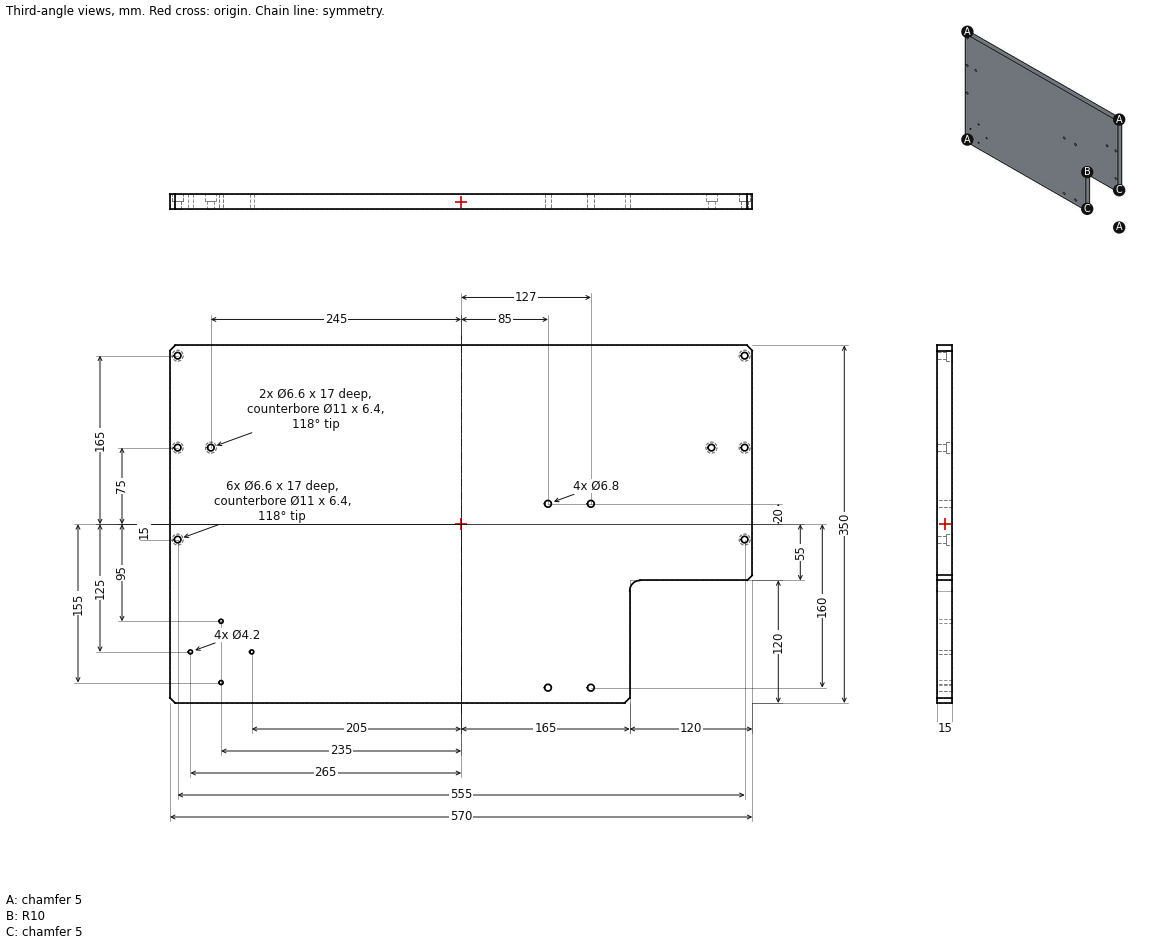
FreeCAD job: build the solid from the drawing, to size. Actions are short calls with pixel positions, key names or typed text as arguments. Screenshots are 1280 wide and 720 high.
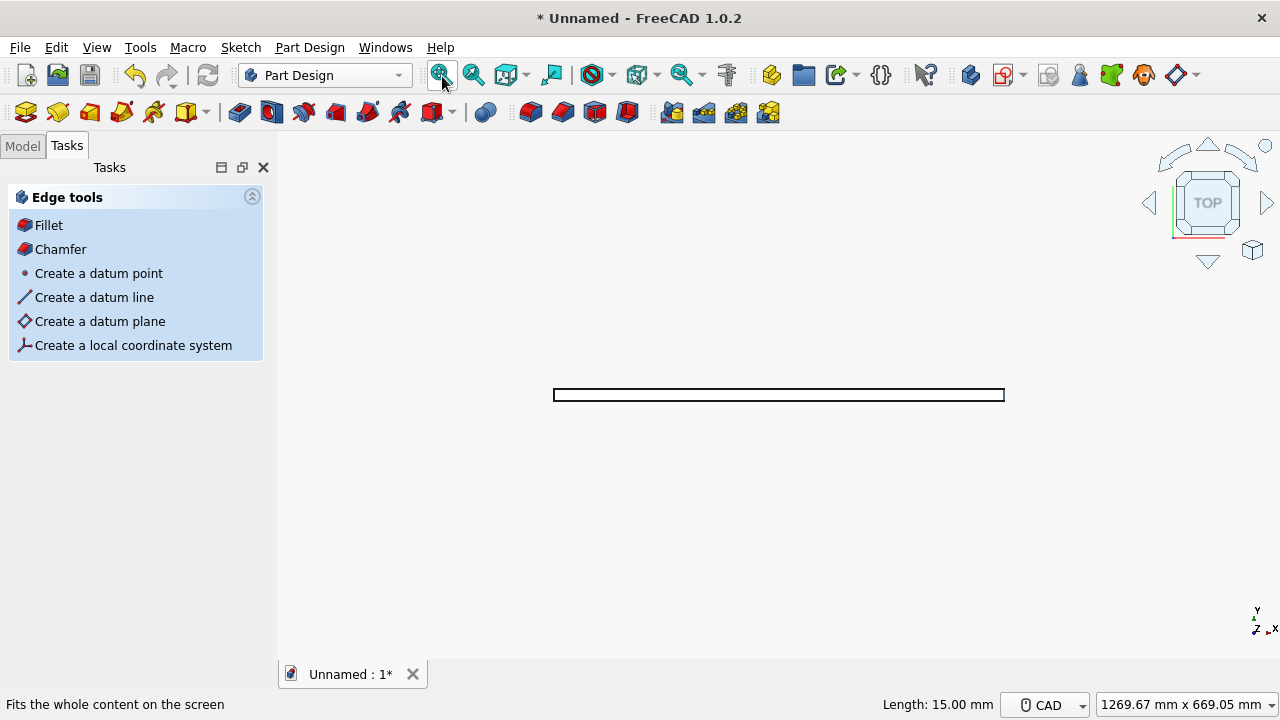
click(442, 76)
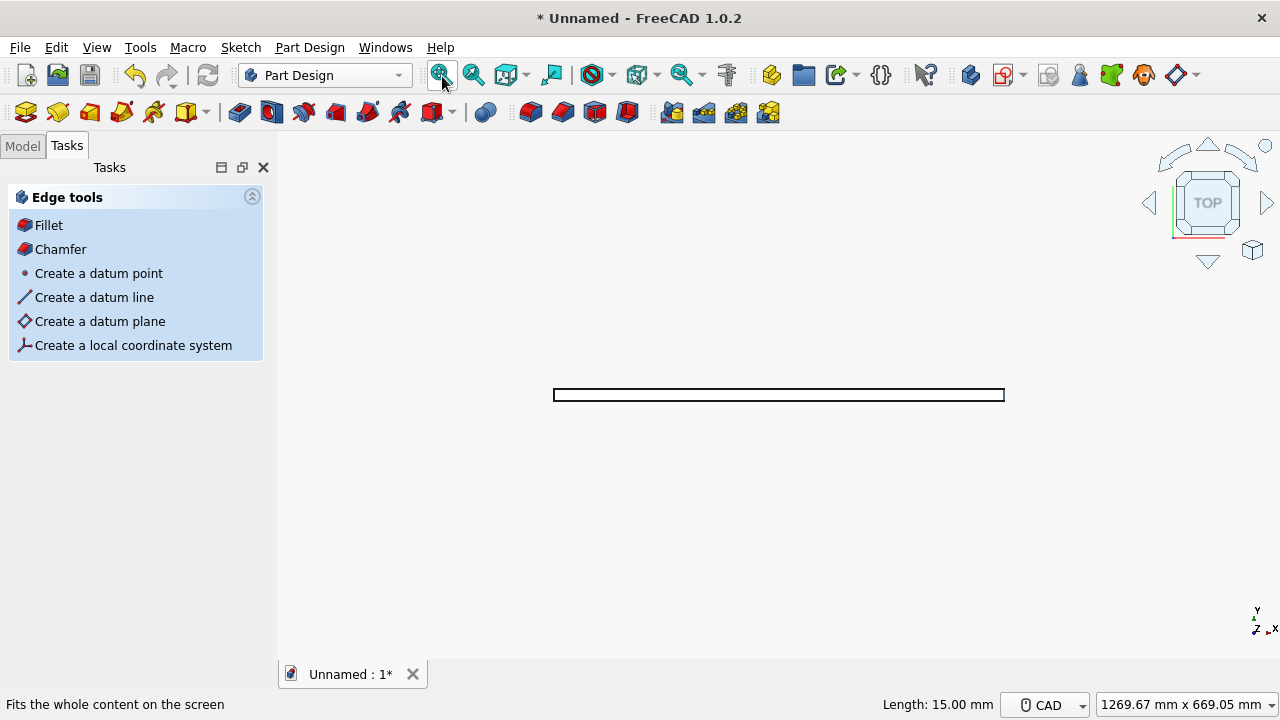
click(554, 395, ctrl)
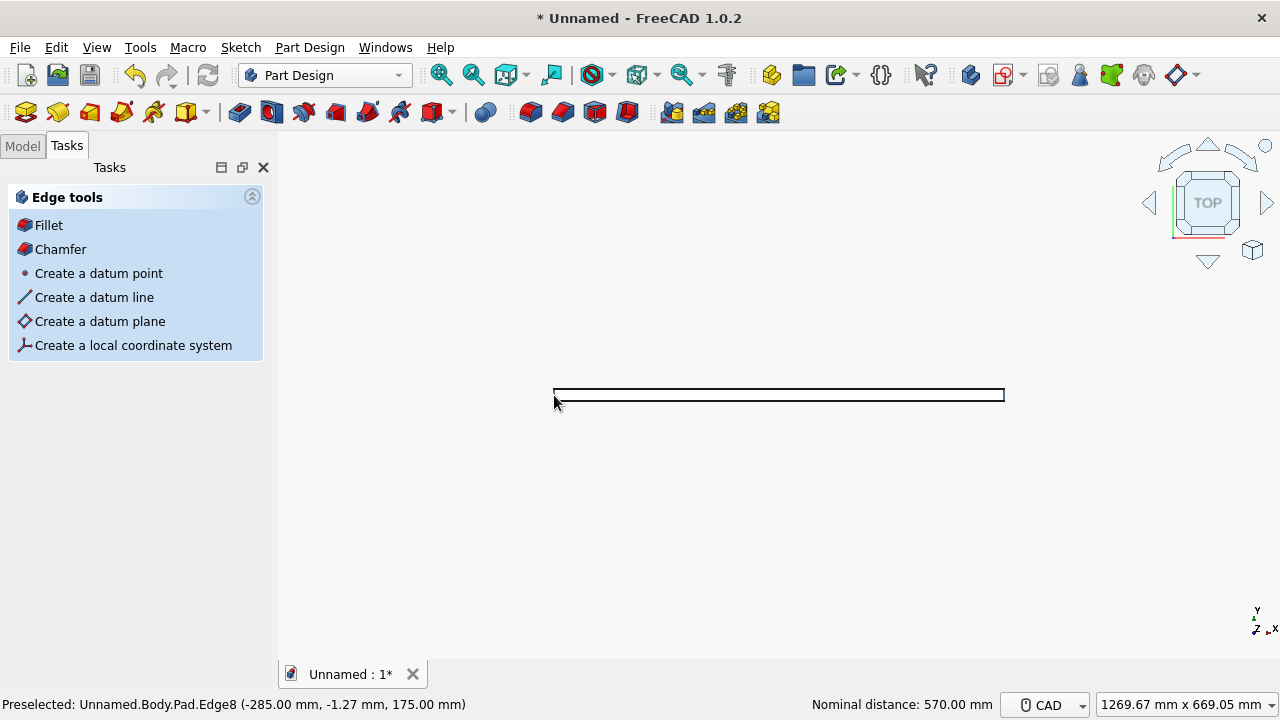
scroll(554, 394, up, 7)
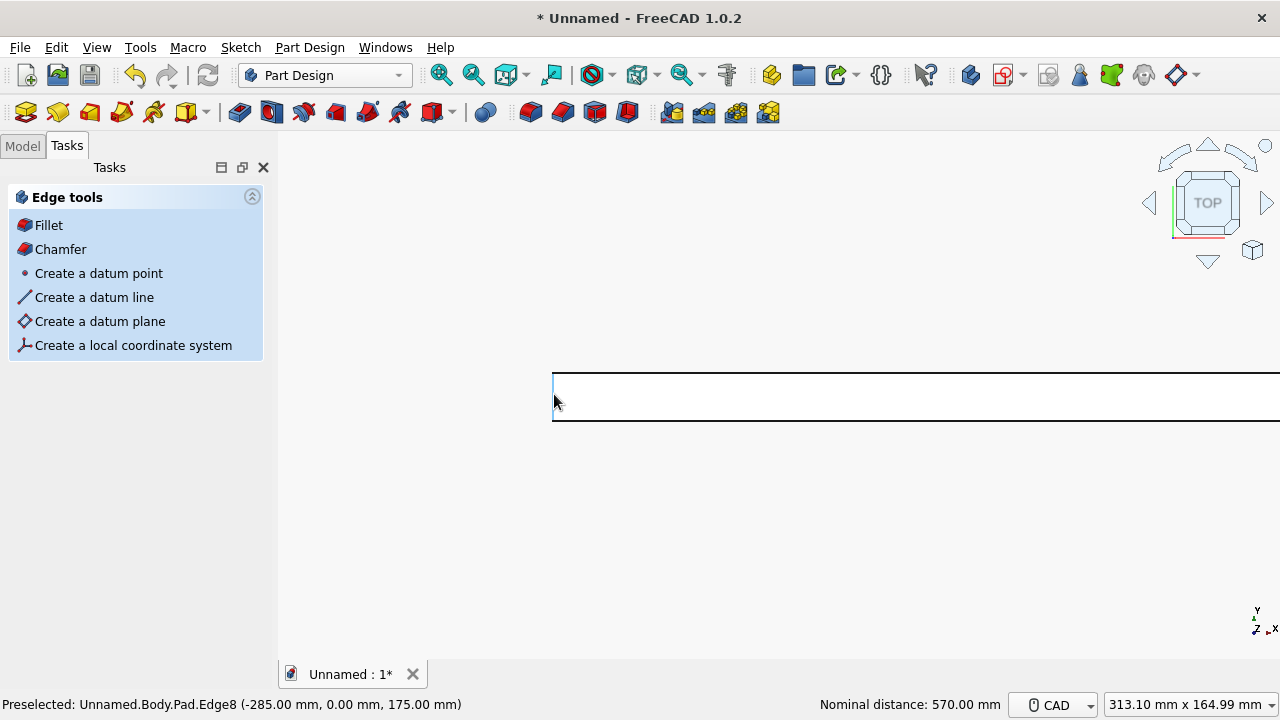
click(442, 76)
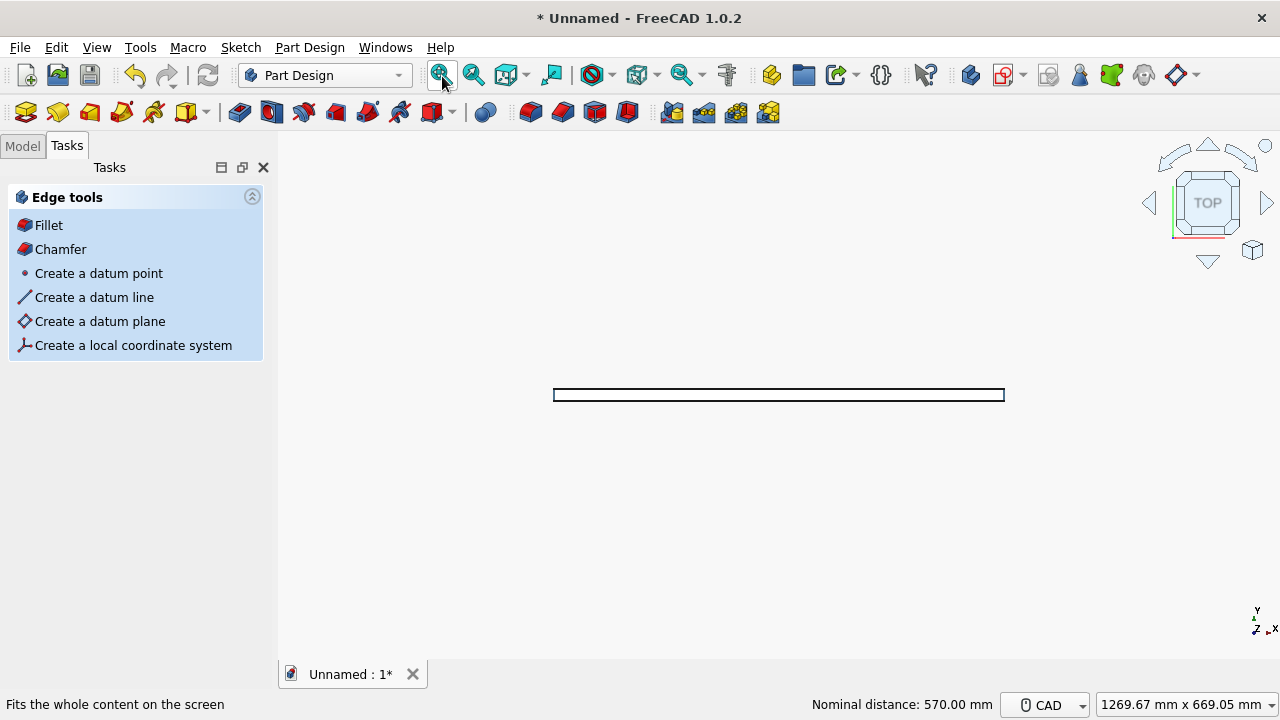
key(1)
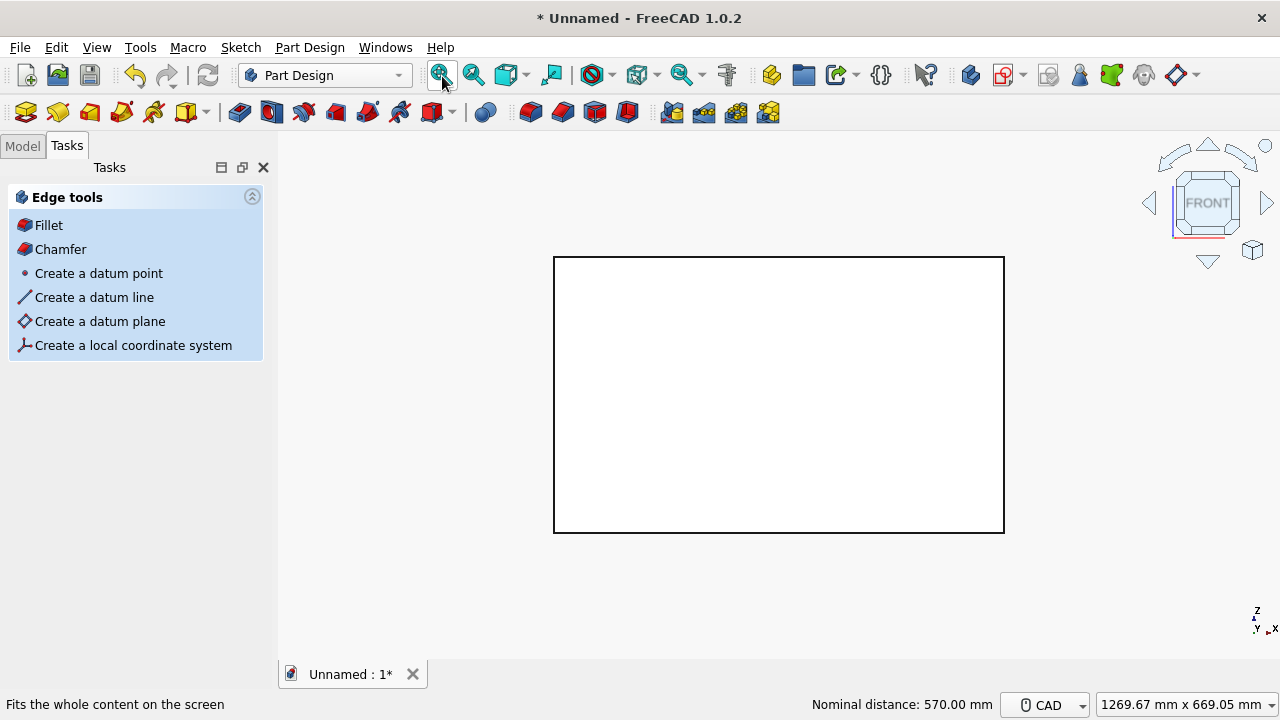
scroll(554, 532, up, 7)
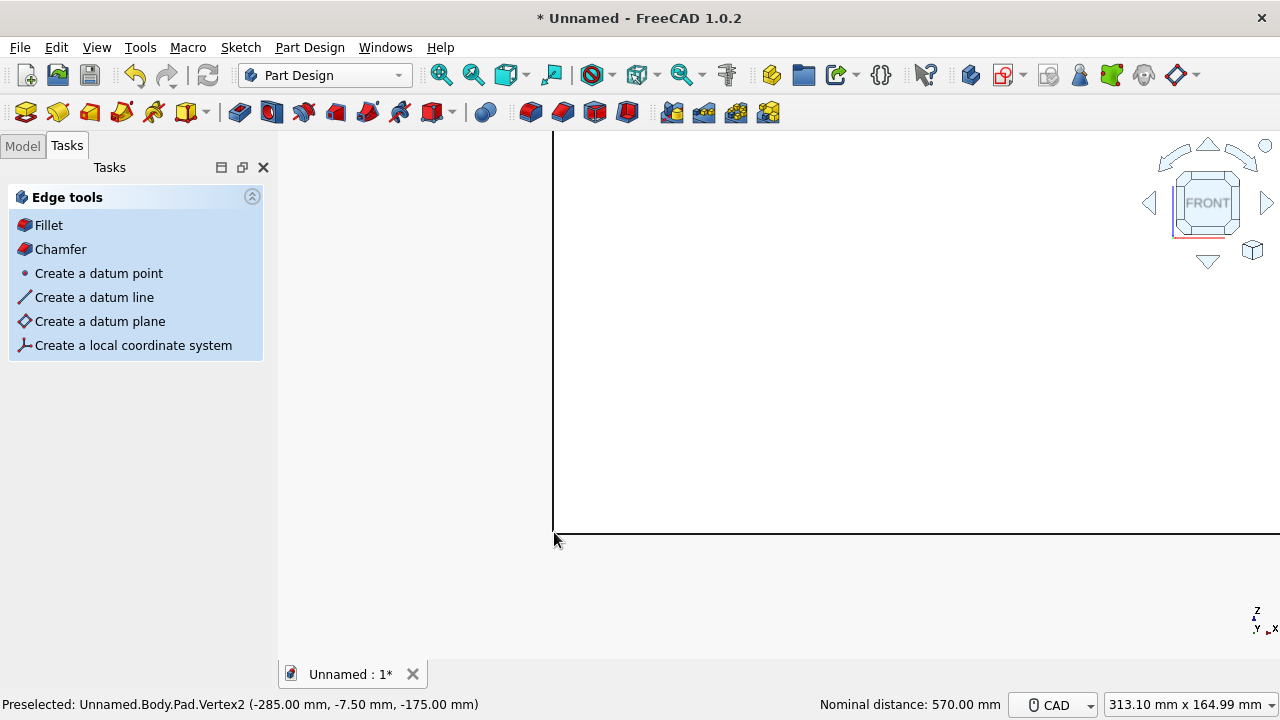
click(442, 76)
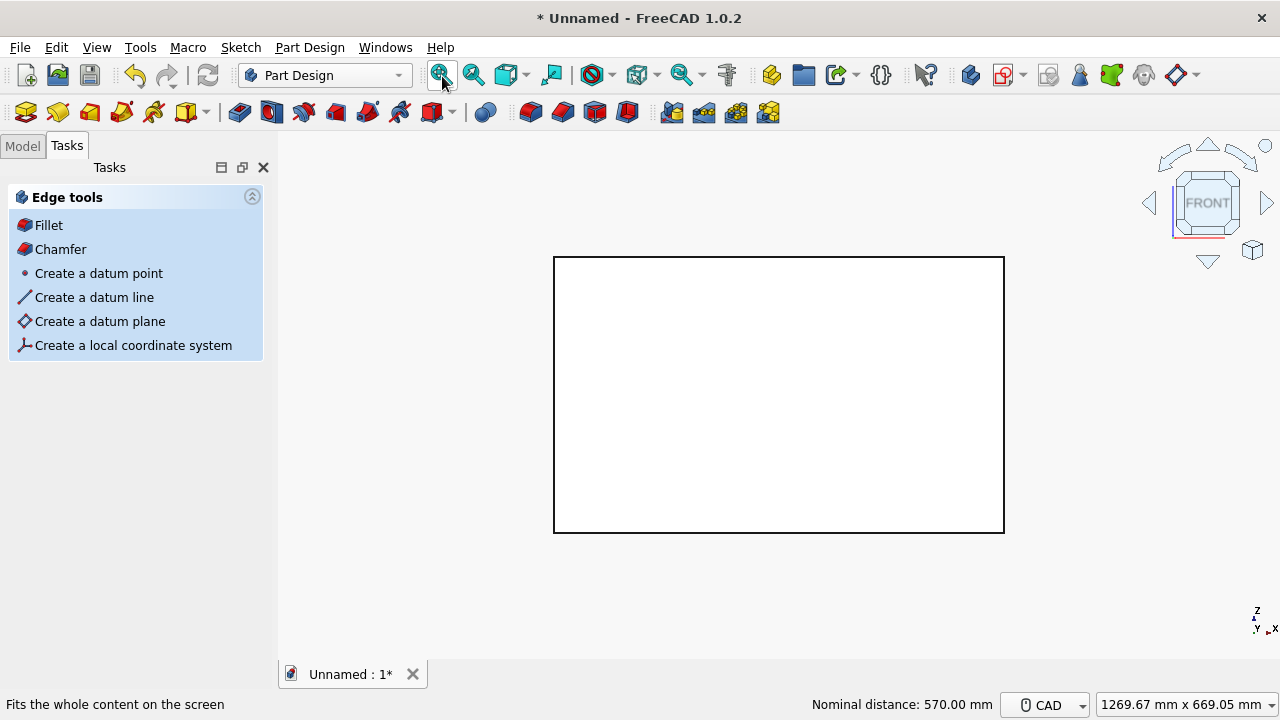
key(3)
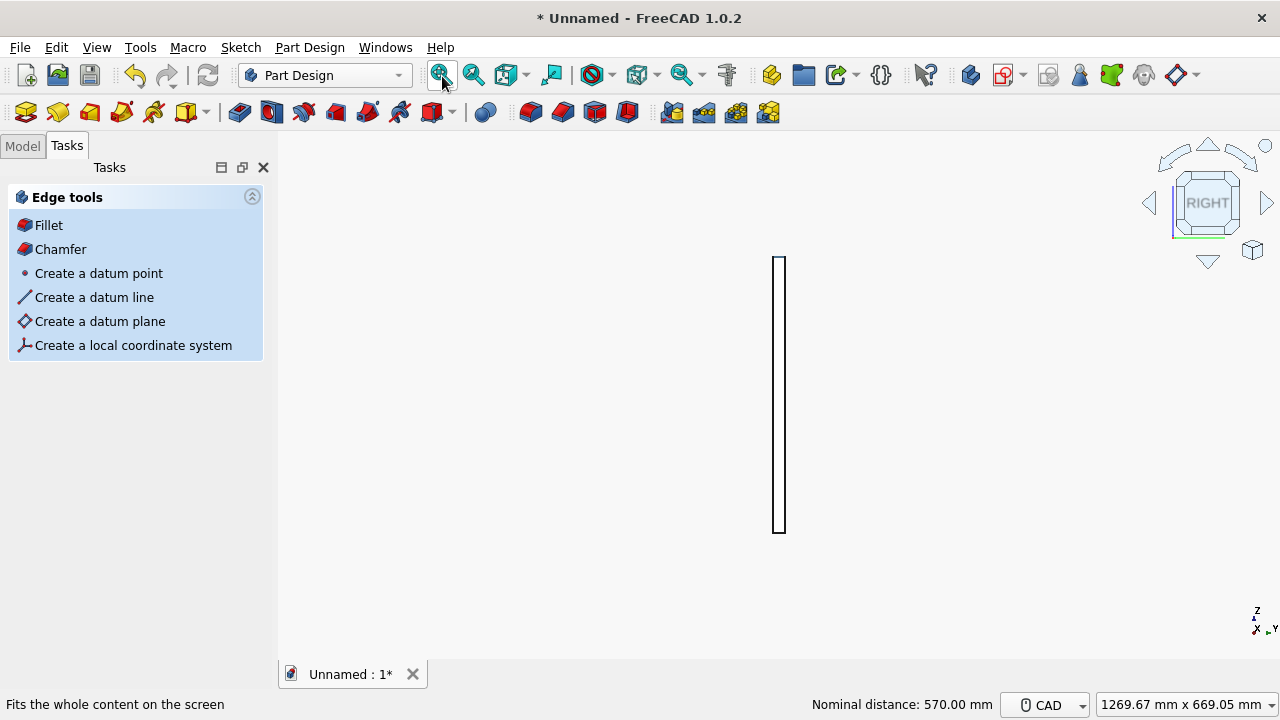
scroll(779, 532, up, 7)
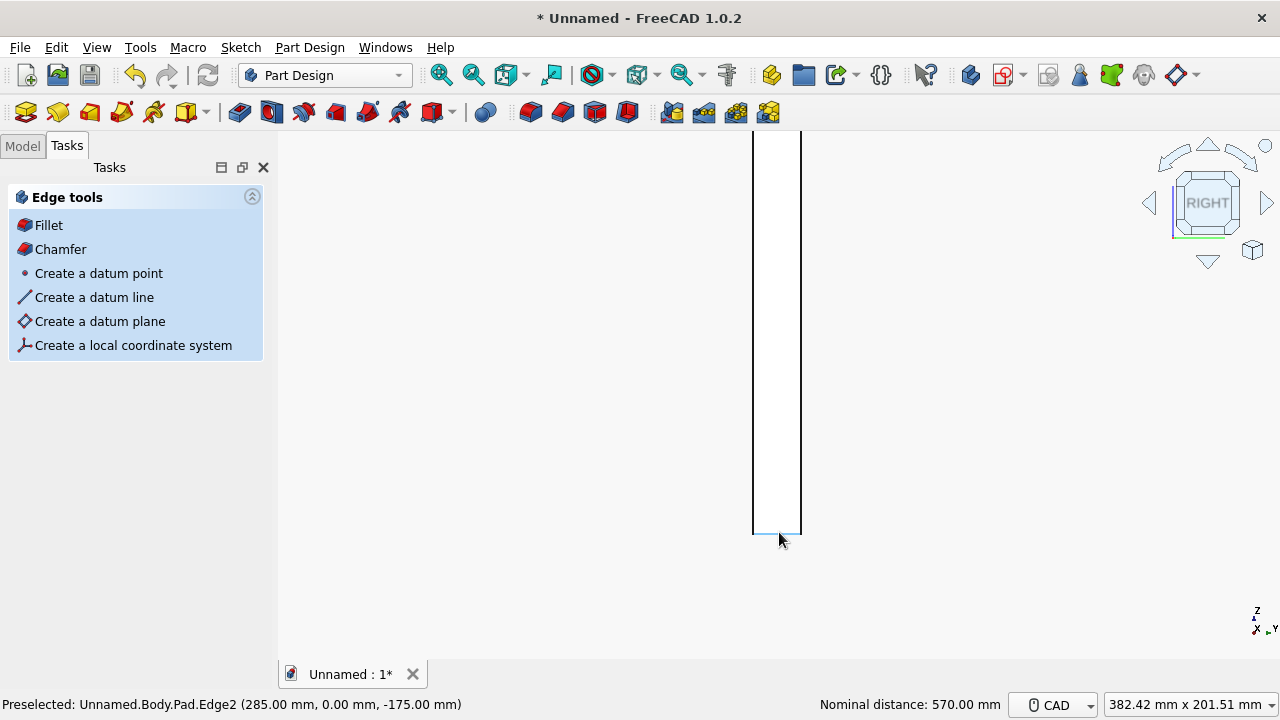
click(777, 533, ctrl)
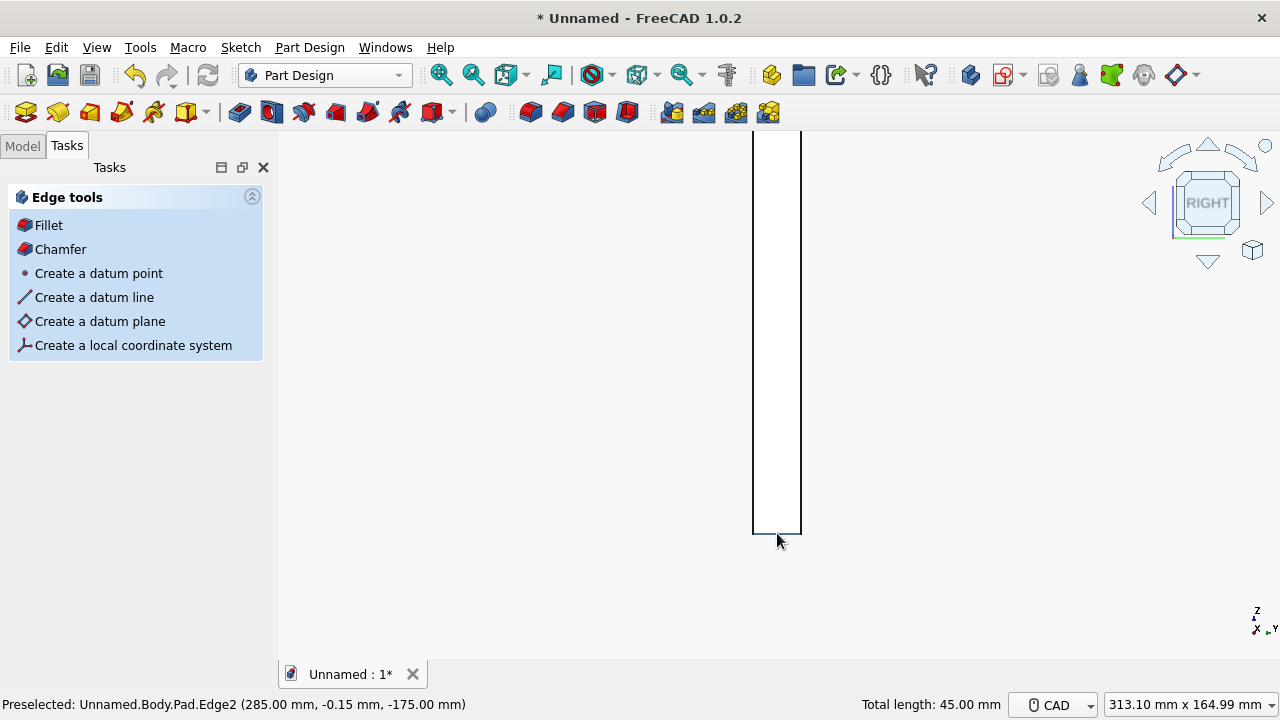
click(442, 76)